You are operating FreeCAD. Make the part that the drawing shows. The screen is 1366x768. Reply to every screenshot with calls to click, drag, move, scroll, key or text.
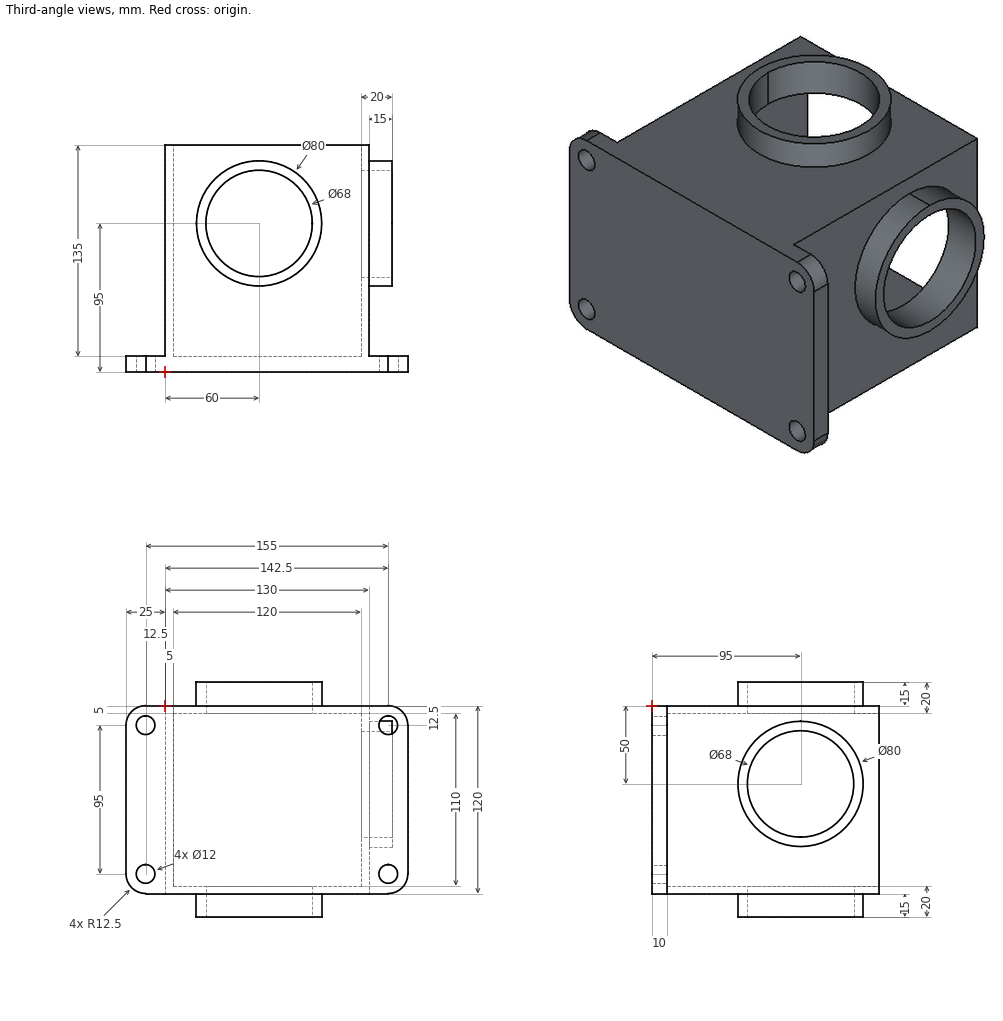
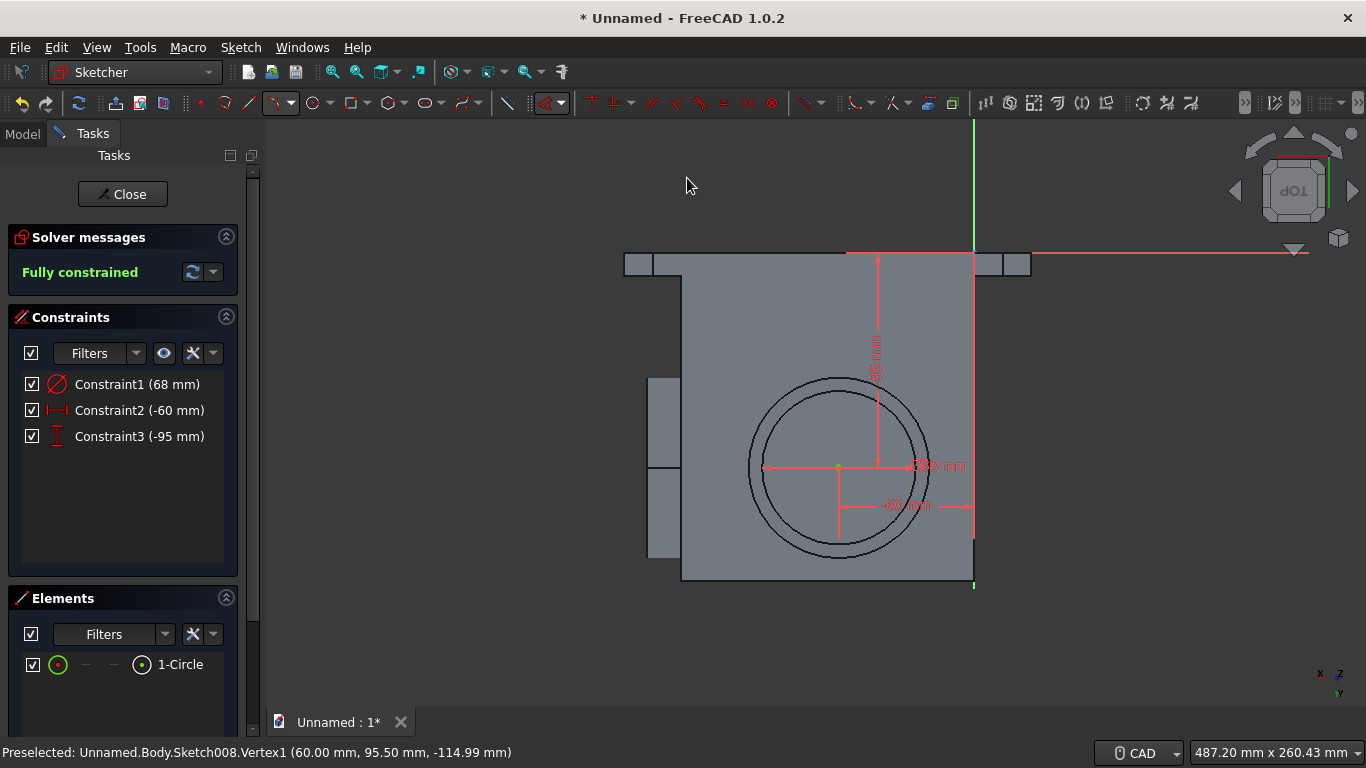
click(123, 194)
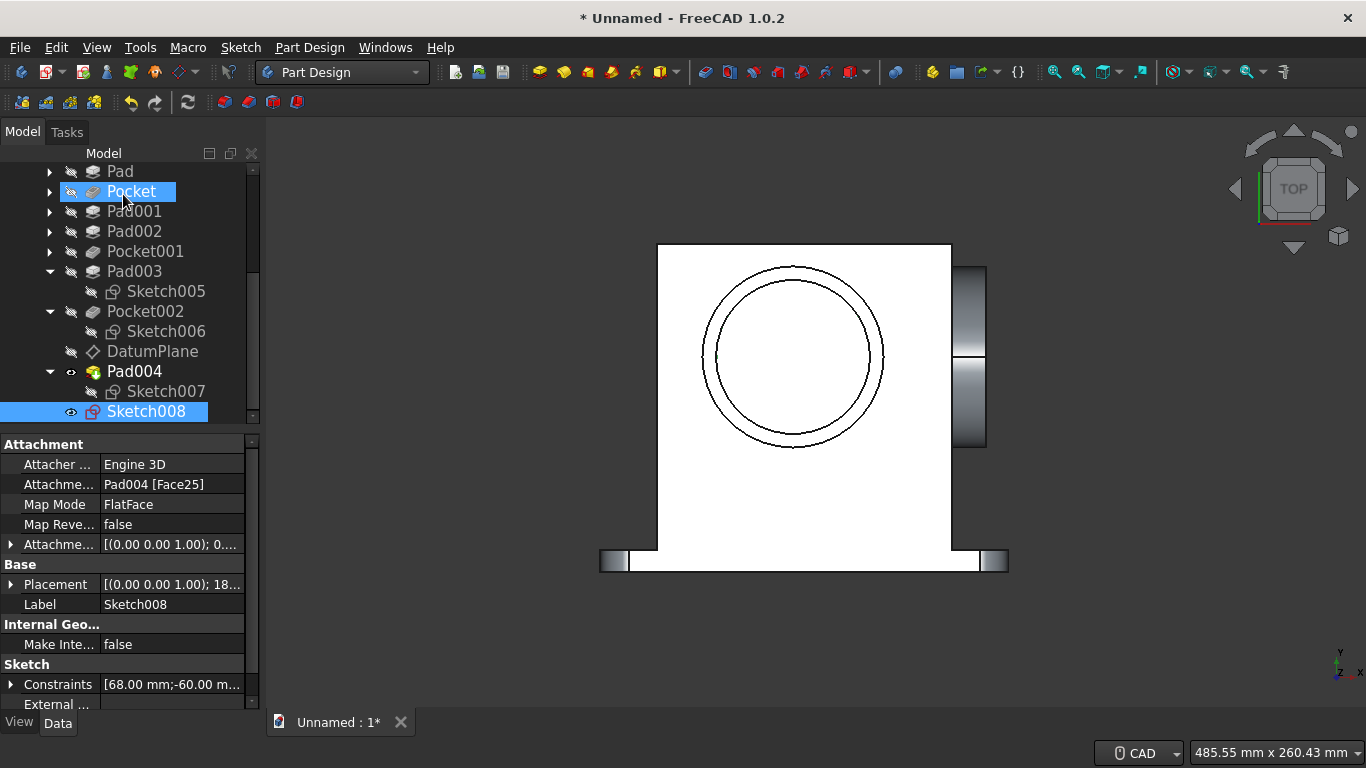
click(706, 72)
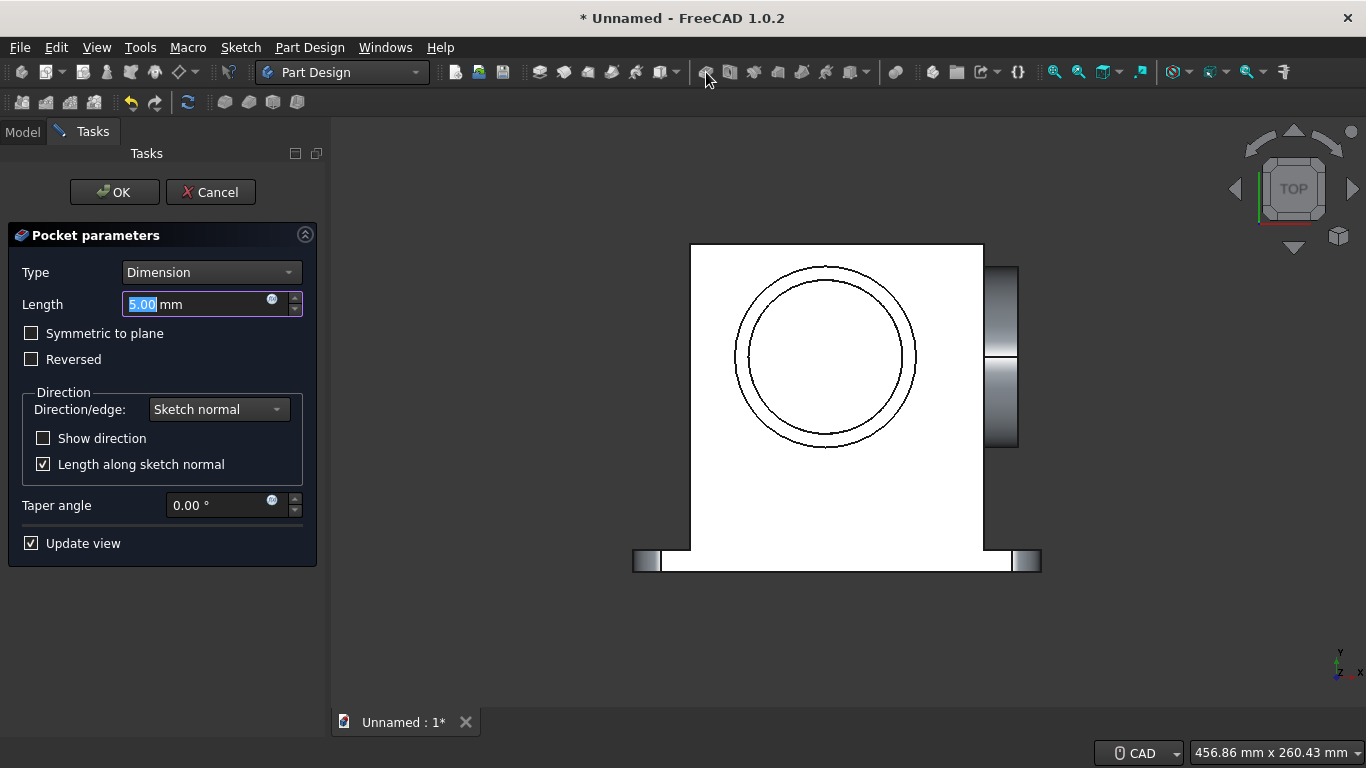
text(20)
key(Tab)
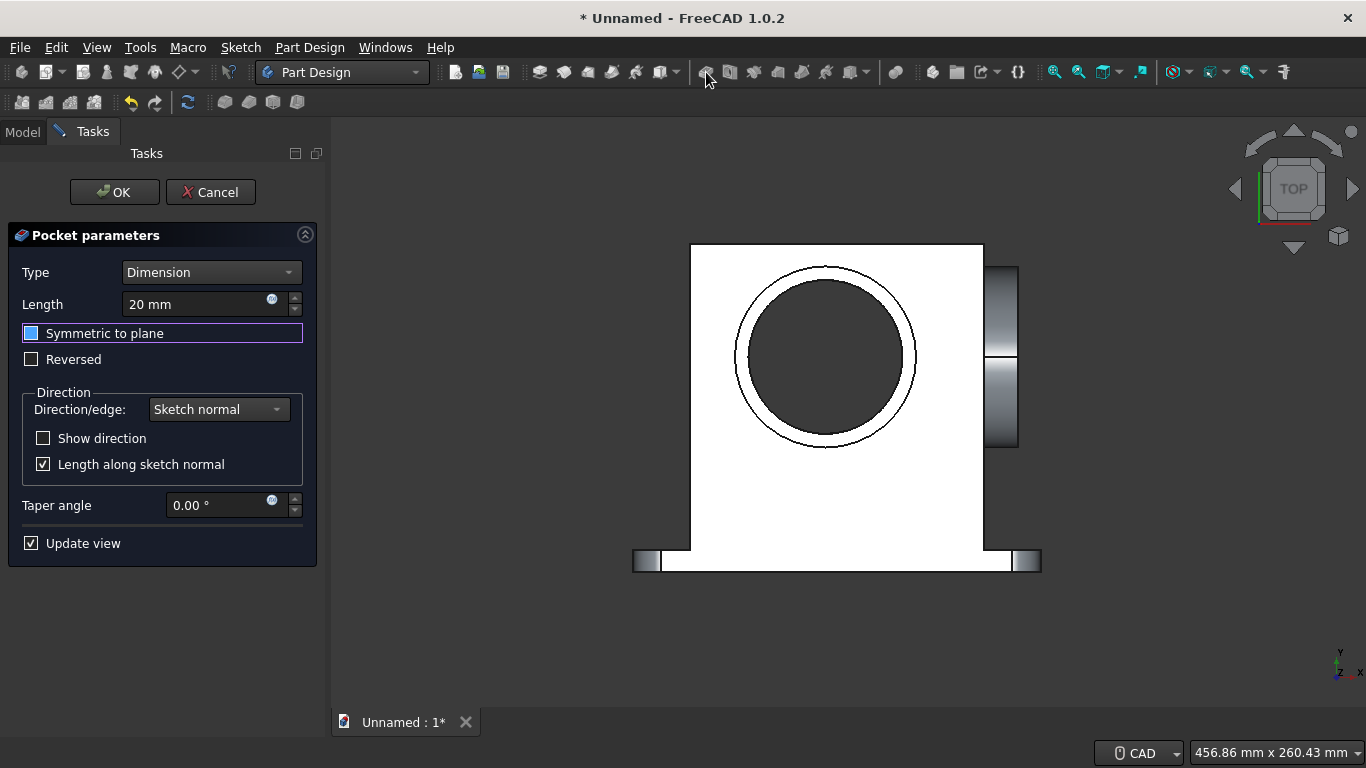
click(115, 192)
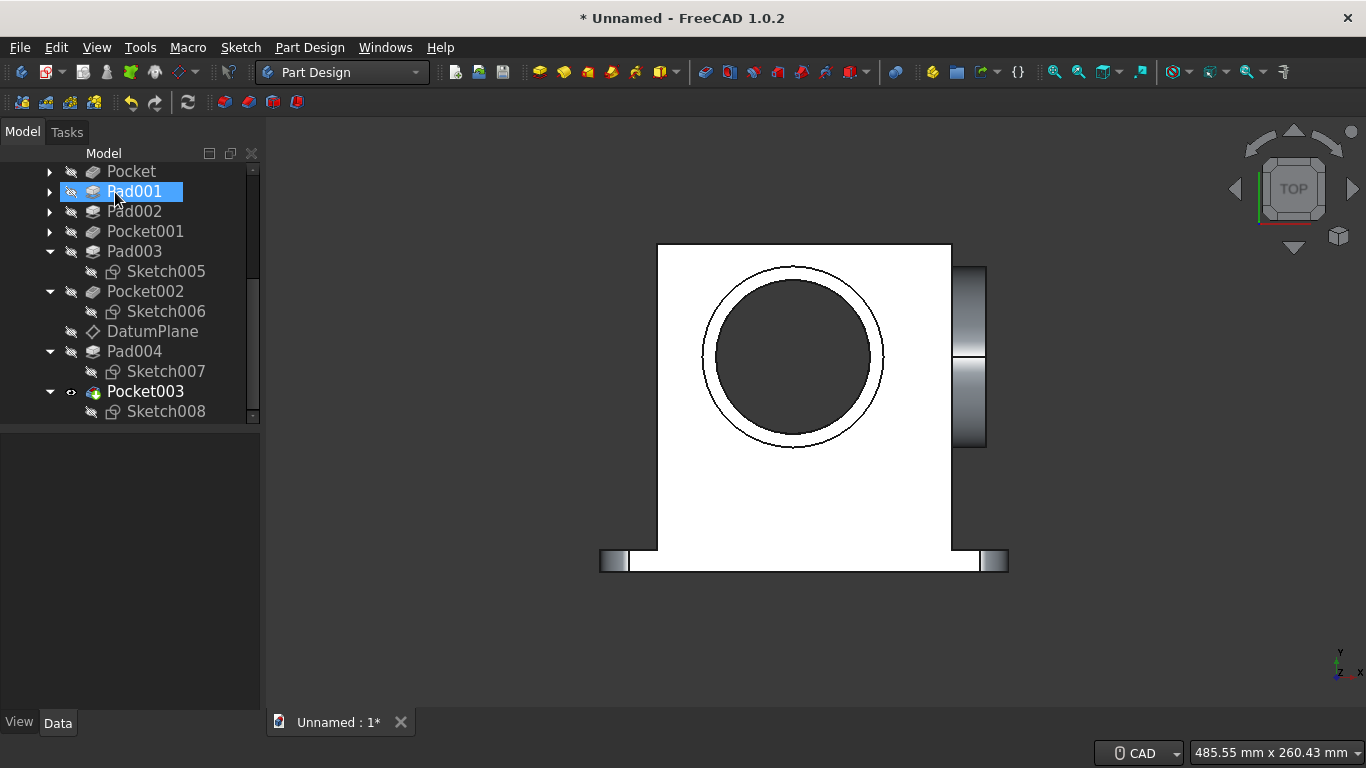
key(0)